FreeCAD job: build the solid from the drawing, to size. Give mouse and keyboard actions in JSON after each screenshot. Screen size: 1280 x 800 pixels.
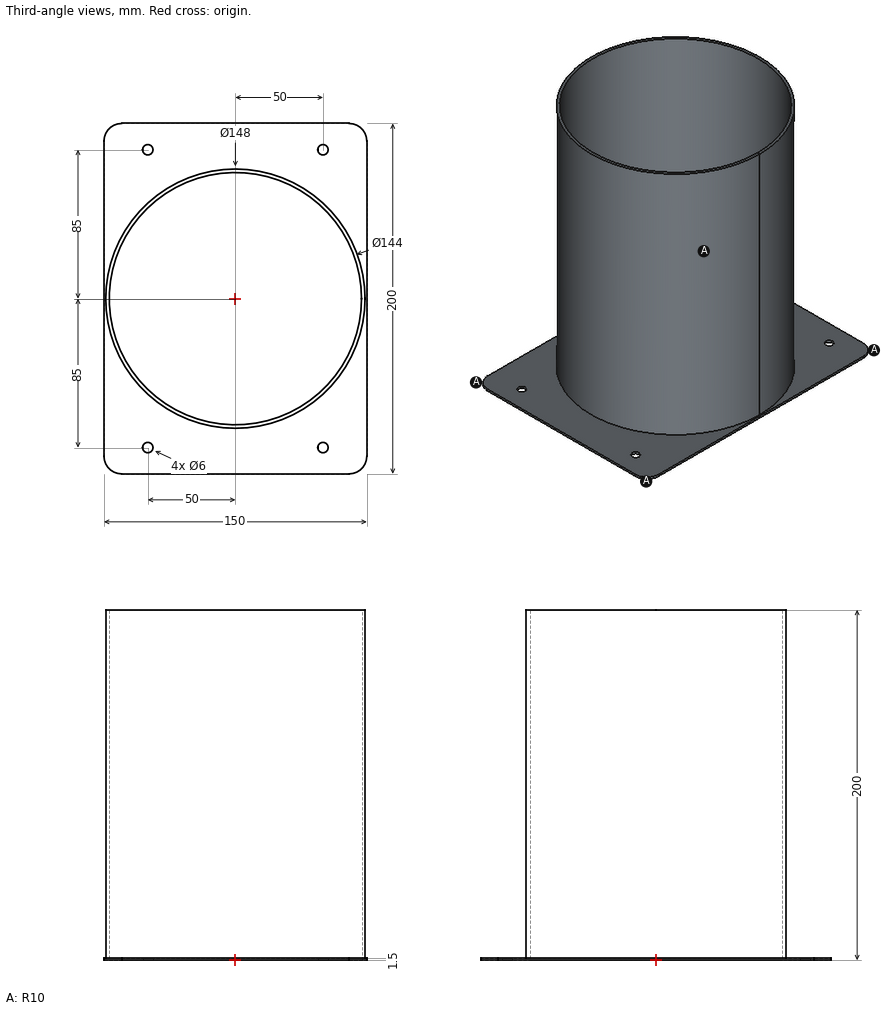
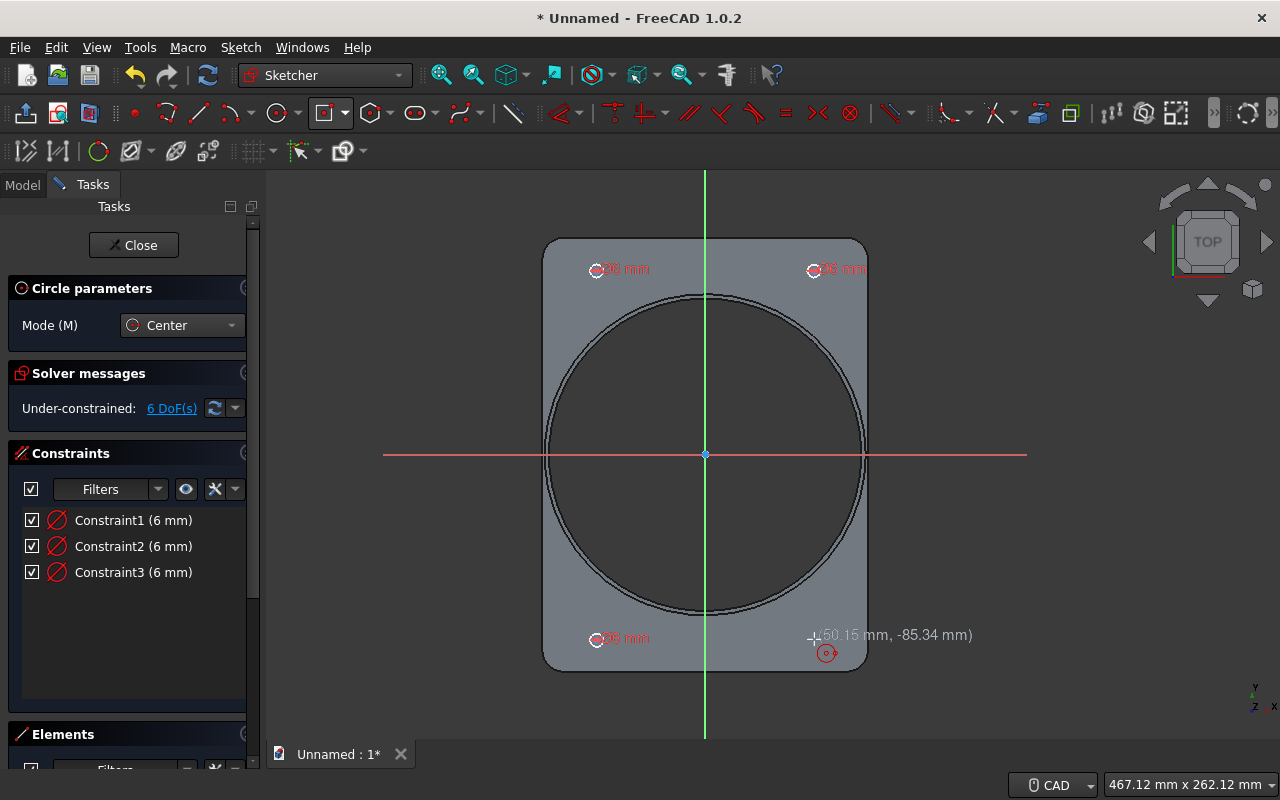
{"action": "left_click", "coordinate": [814, 639]}
{"action": "mouse_move", "coordinate": [818, 635]}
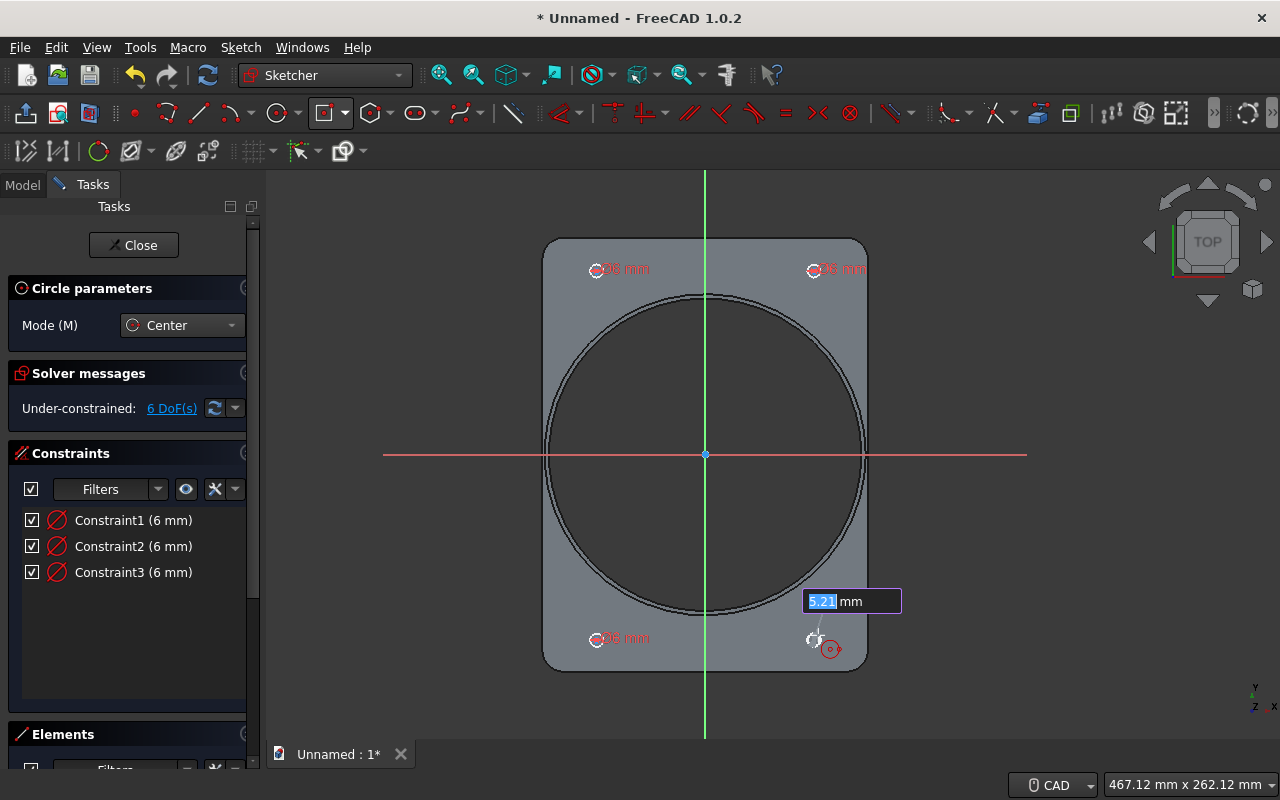
{"action": "type", "text": "6"}
{"action": "key", "text": "Return"}
{"action": "key", "text": "Escape"}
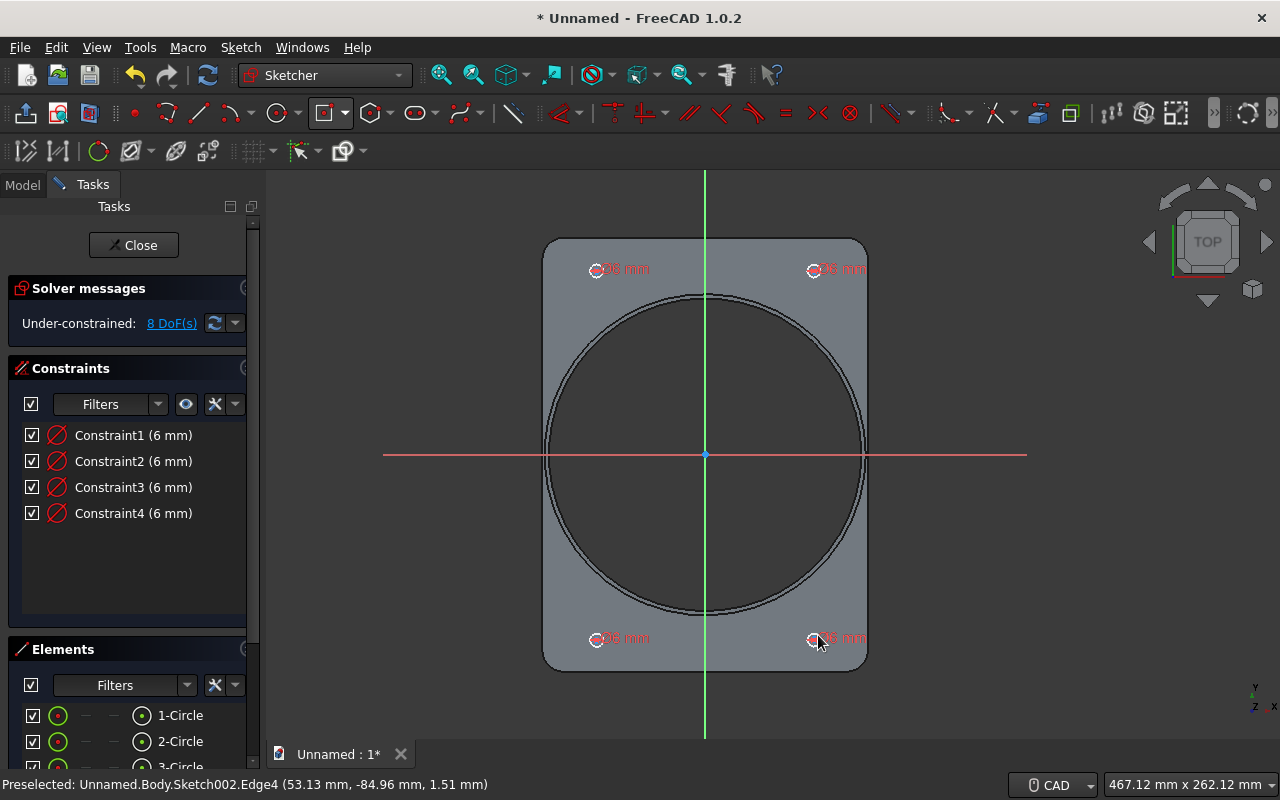
{"action": "left_click", "coordinate": [597, 640]}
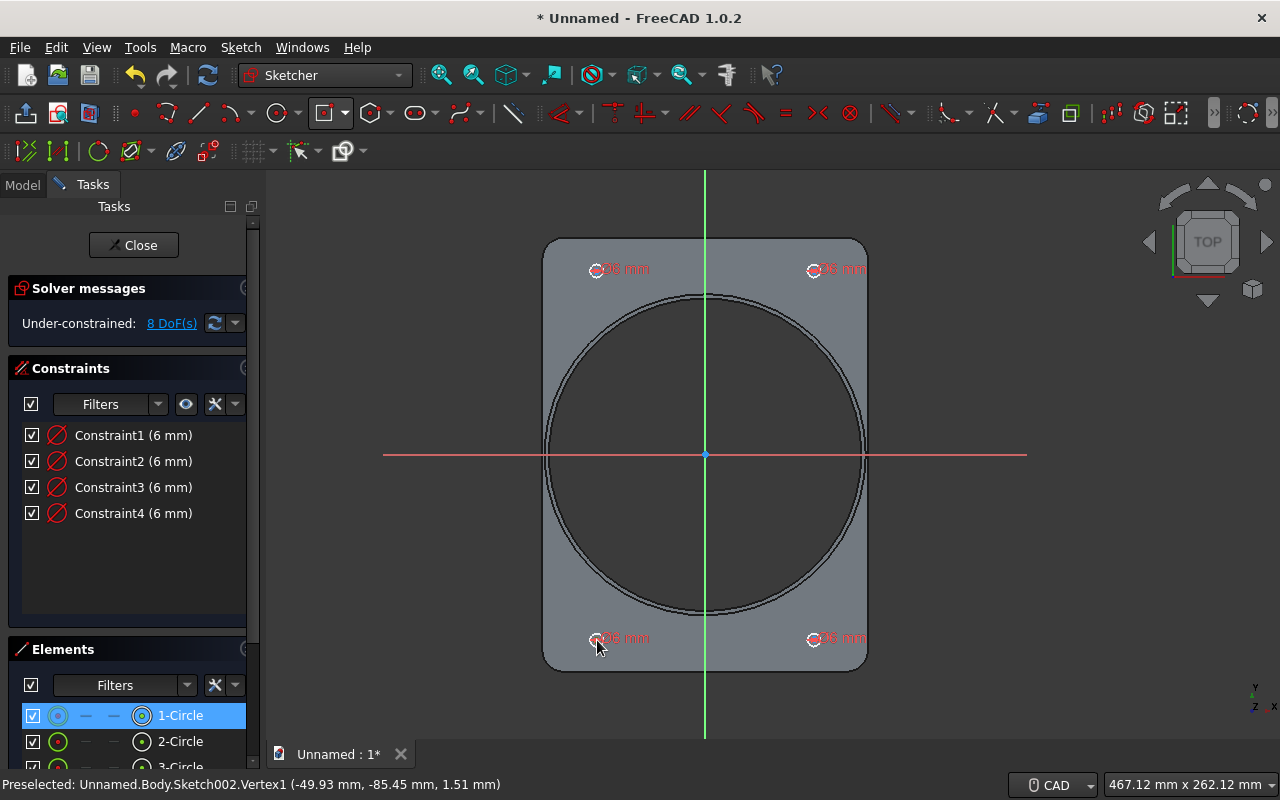
{"action": "left_click", "coordinate": [597, 271]}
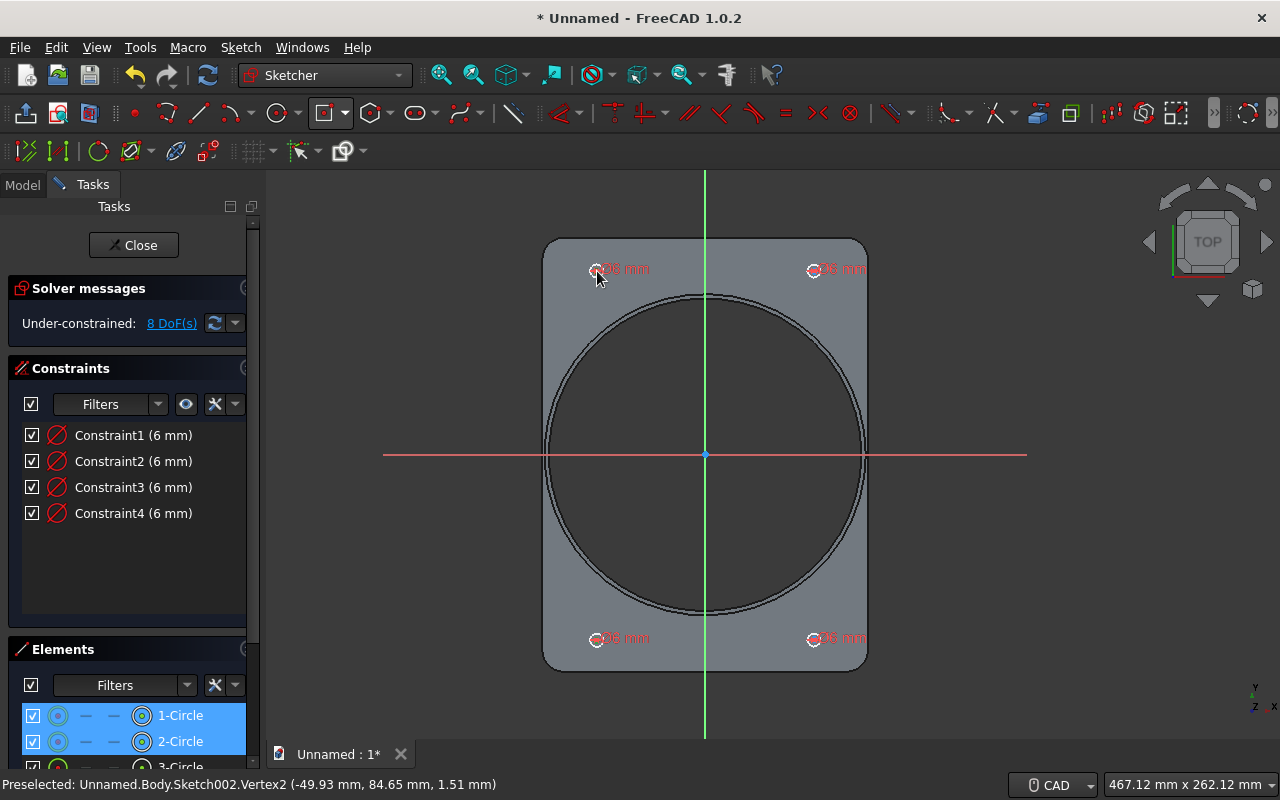
{"action": "left_click", "coordinate": [668, 114]}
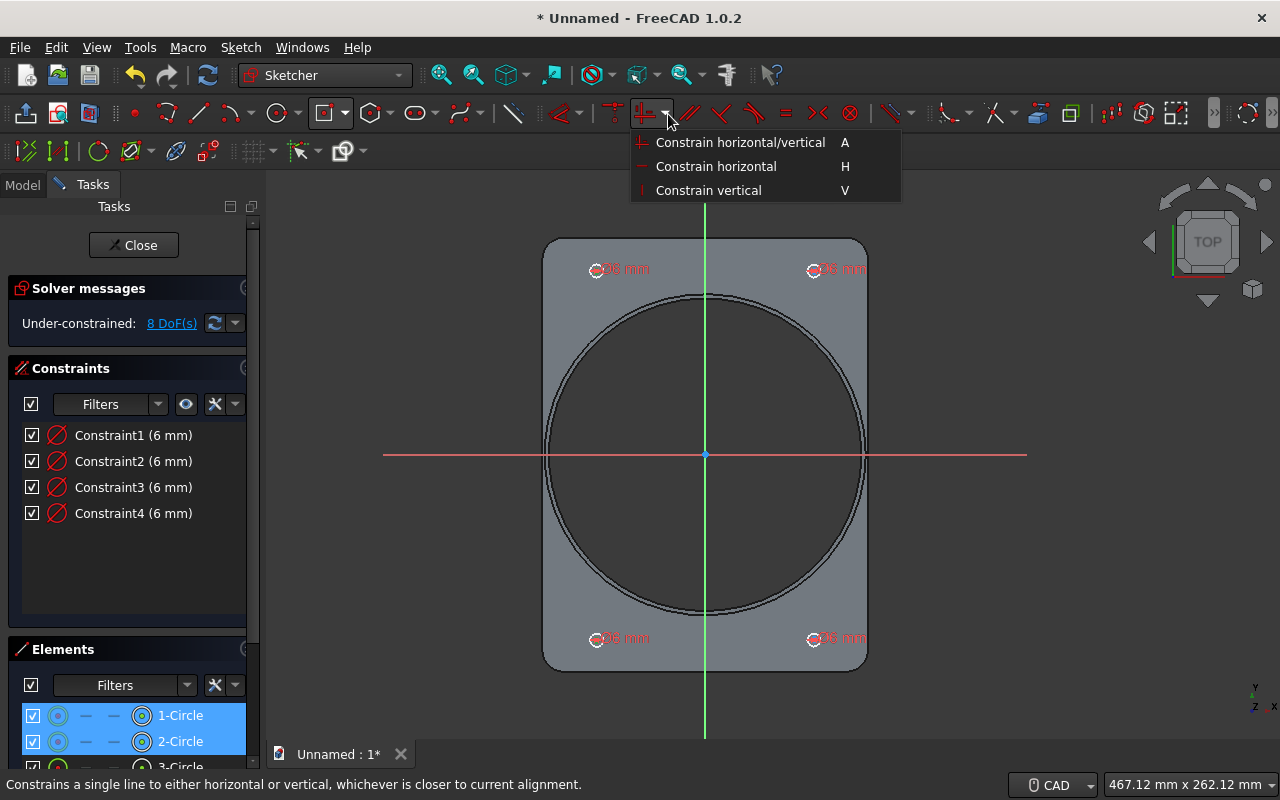
{"action": "left_click", "coordinate": [766, 190]}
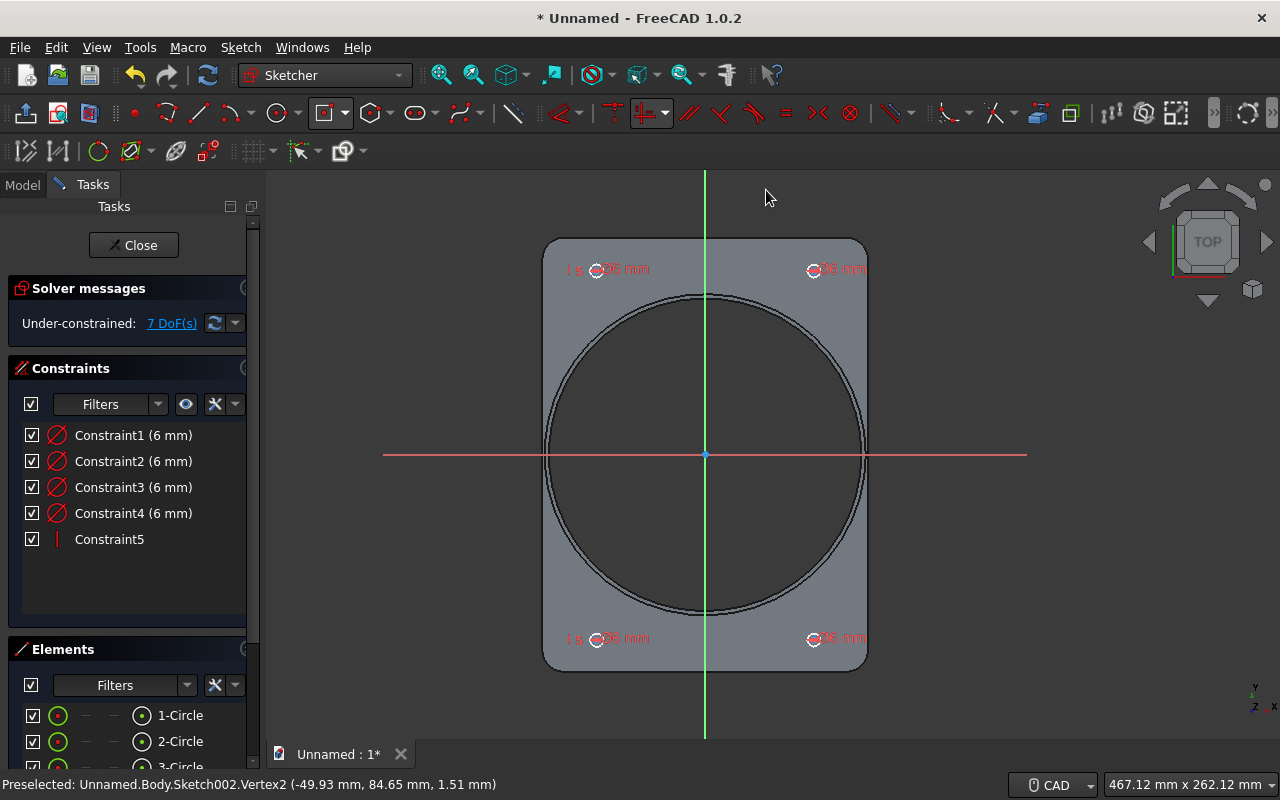
{"action": "left_click", "coordinate": [597, 271]}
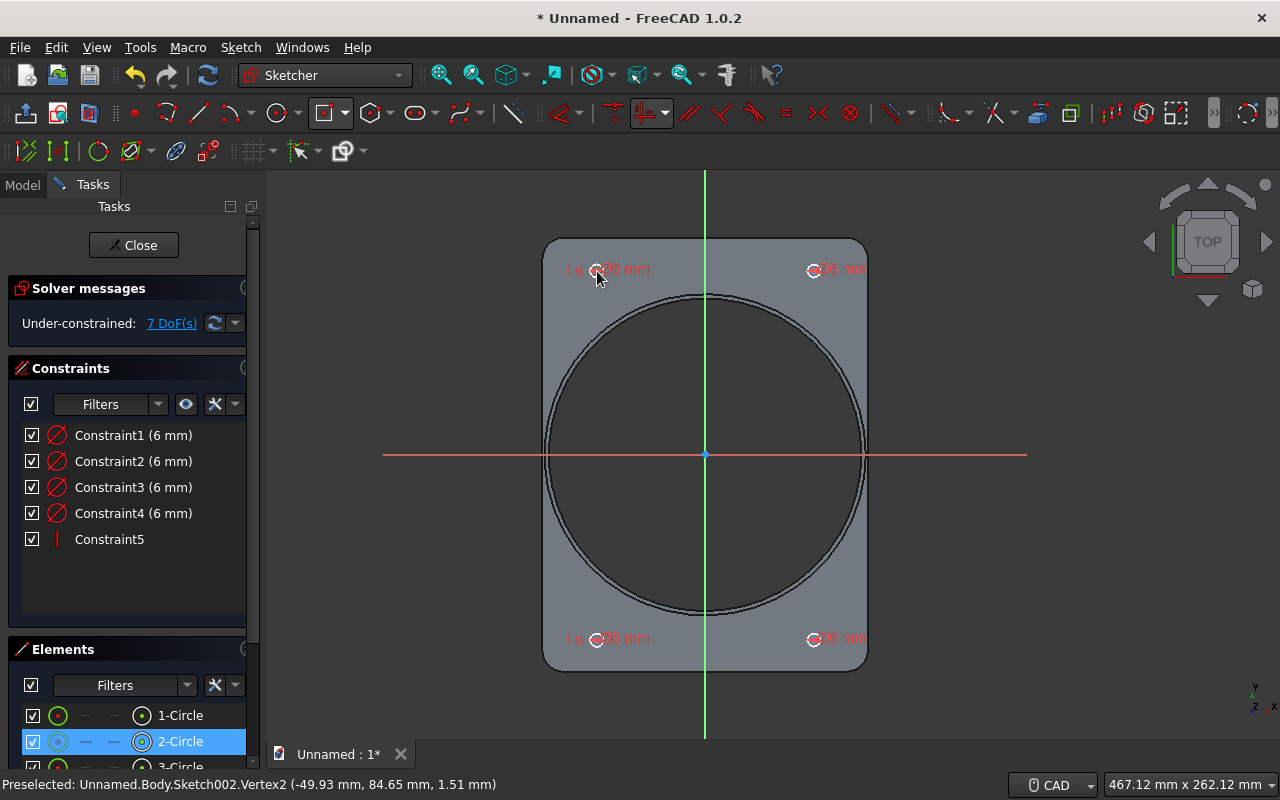
{"action": "left_click", "coordinate": [814, 271]}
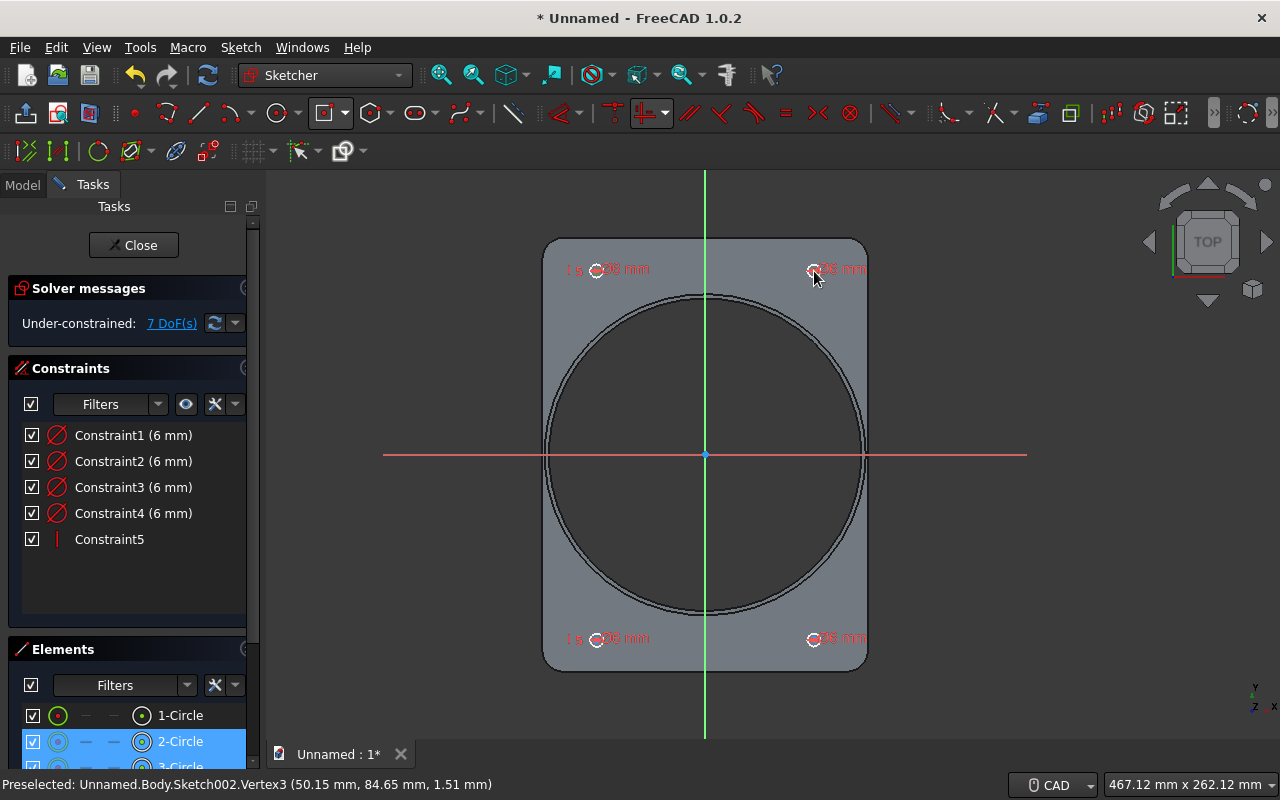
{"action": "left_click", "coordinate": [668, 114]}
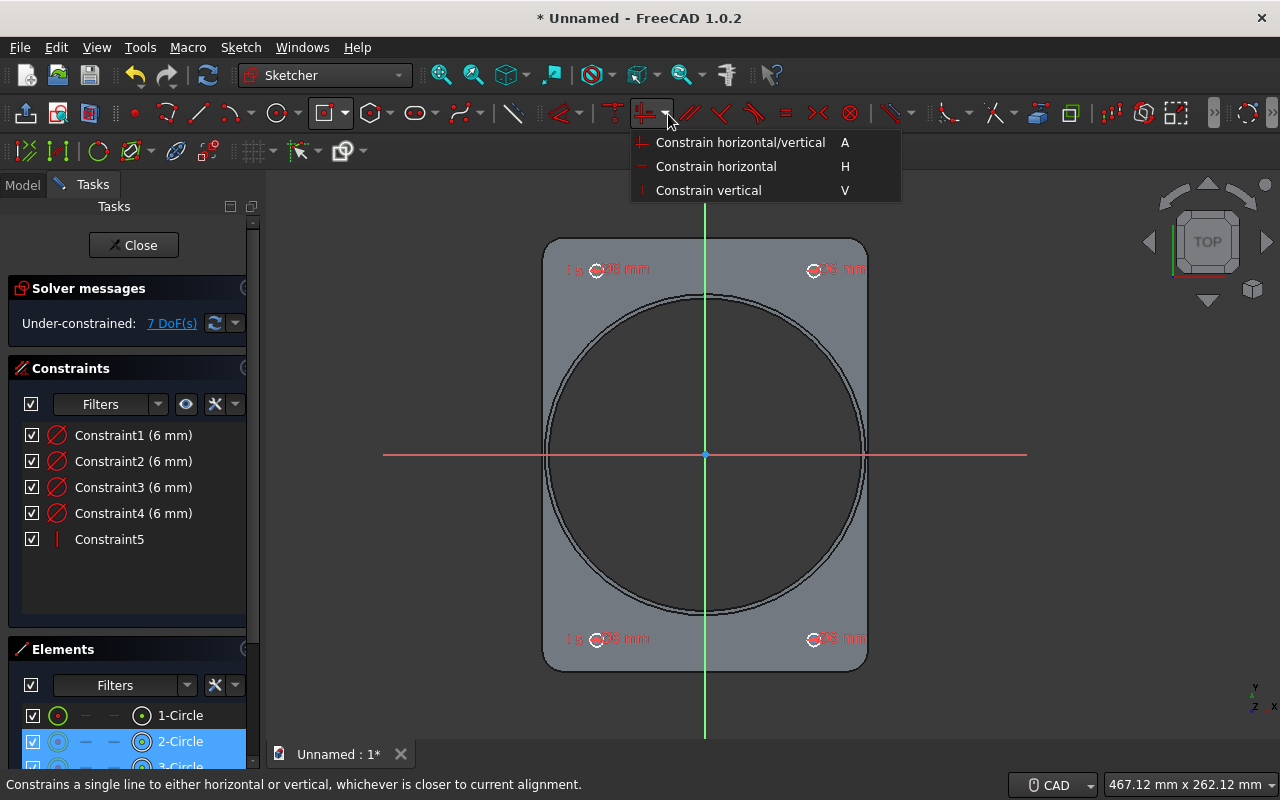
{"action": "left_click", "coordinate": [766, 166]}